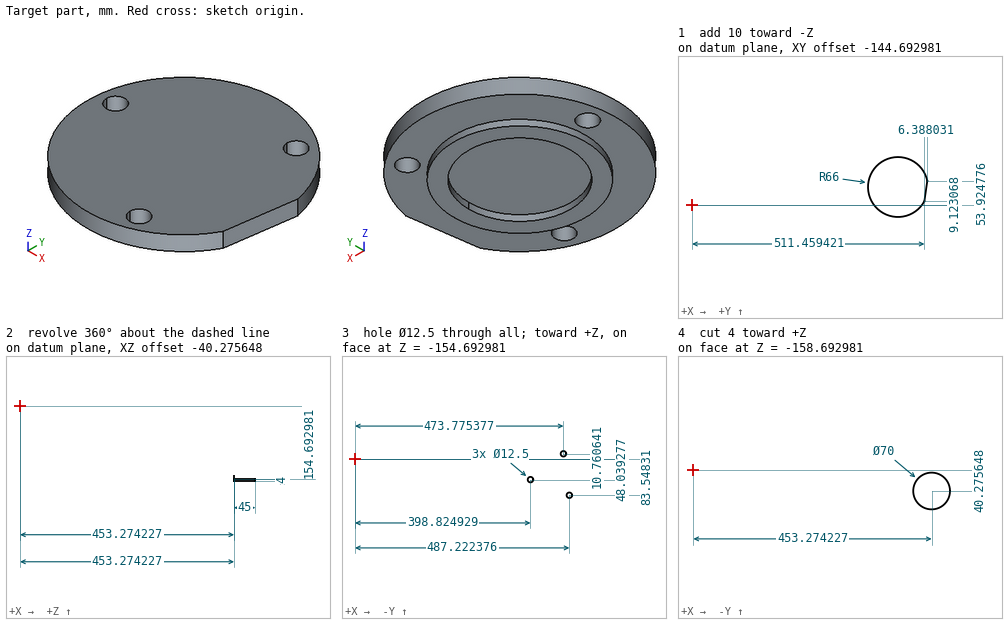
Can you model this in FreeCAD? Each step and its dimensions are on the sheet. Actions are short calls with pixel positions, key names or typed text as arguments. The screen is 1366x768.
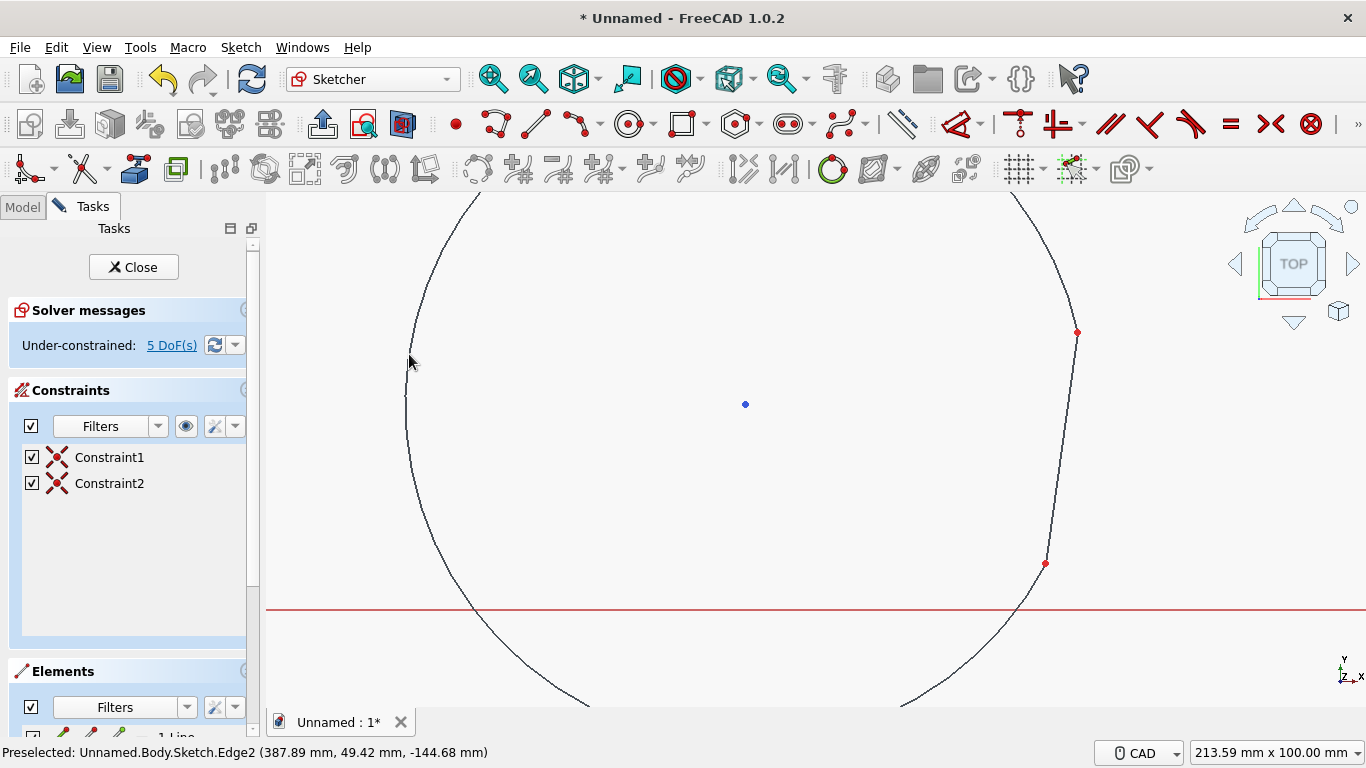
click(409, 358)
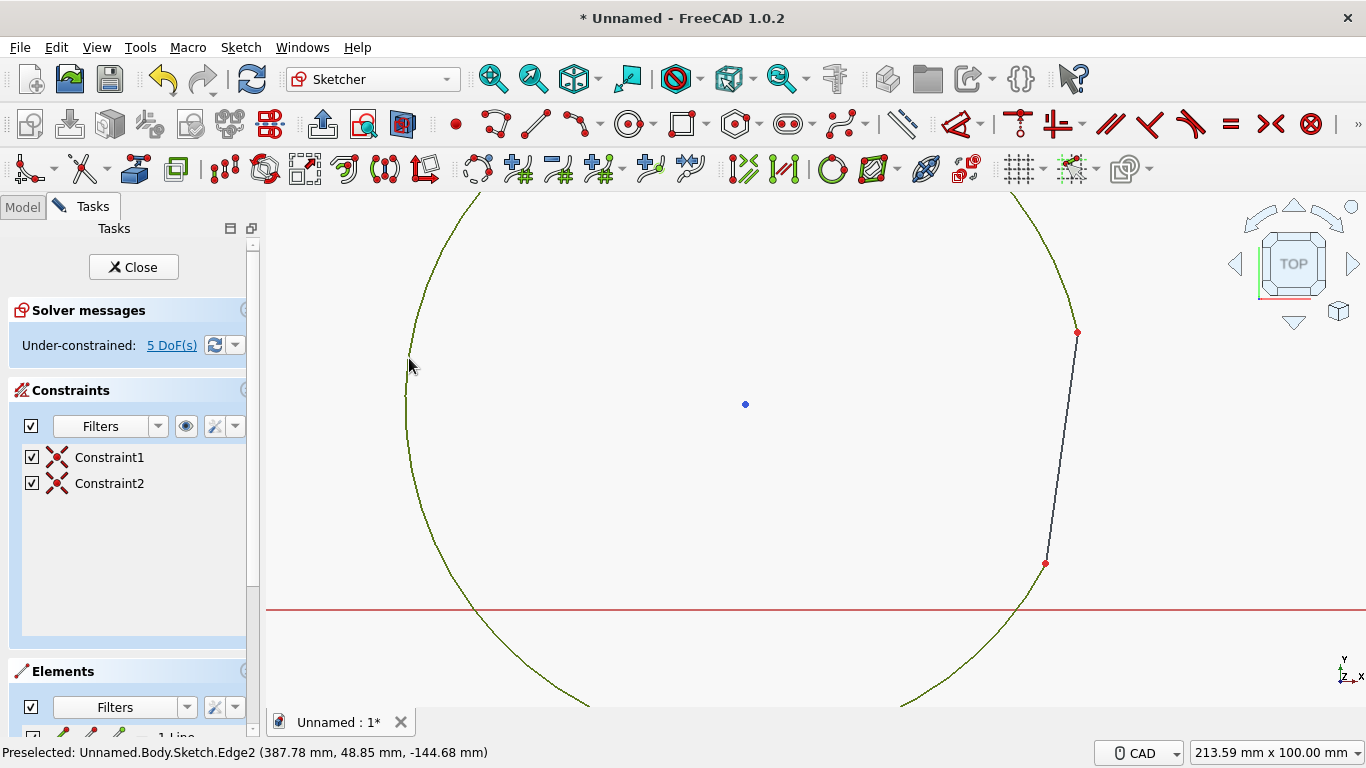
click(982, 124)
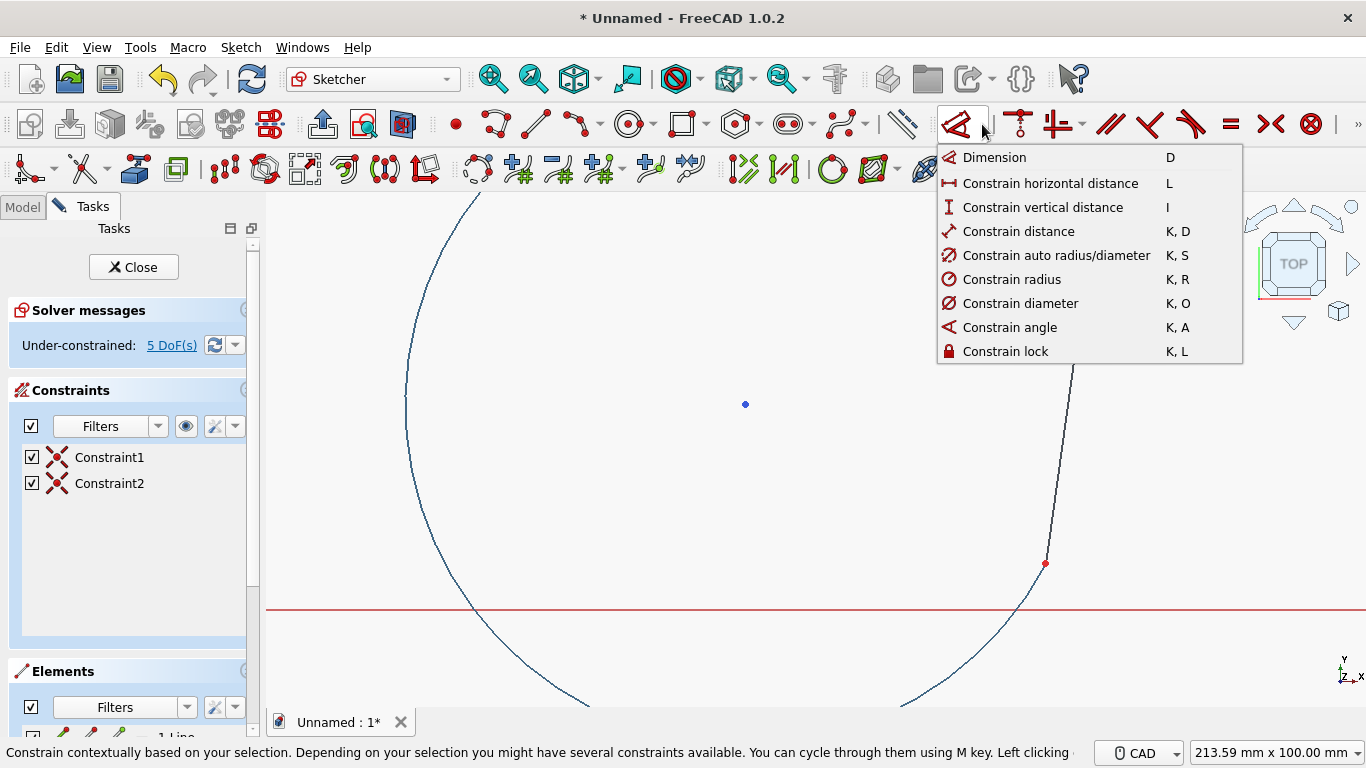
click(1090, 279)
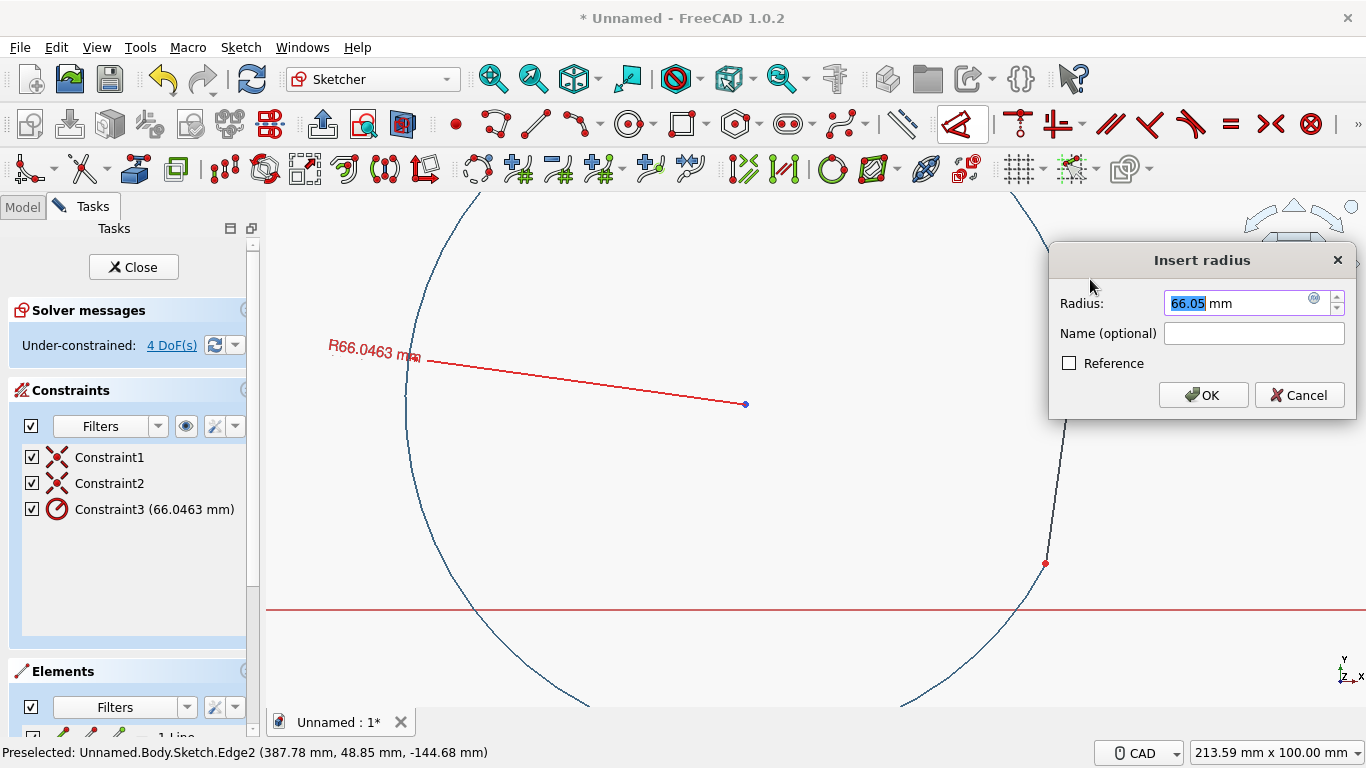
text(66)
key(Return)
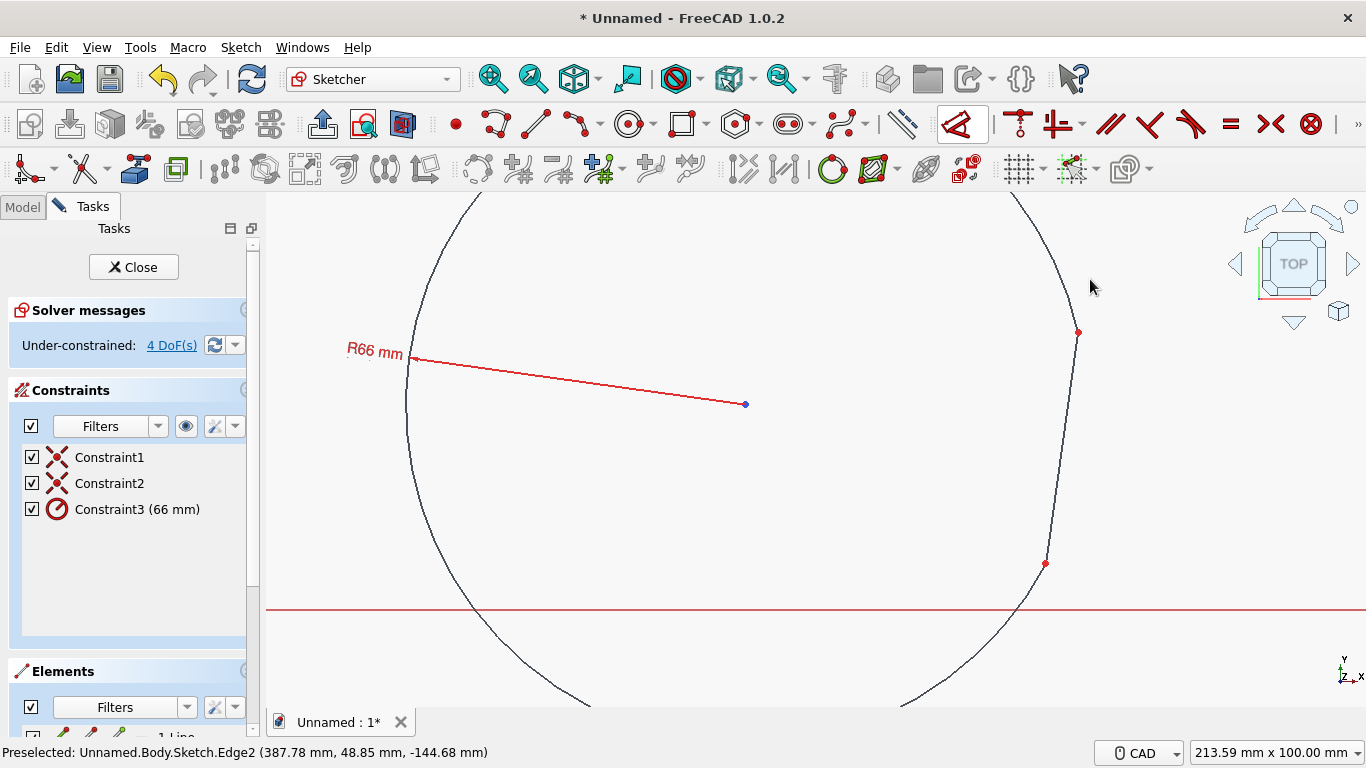
click(1046, 564)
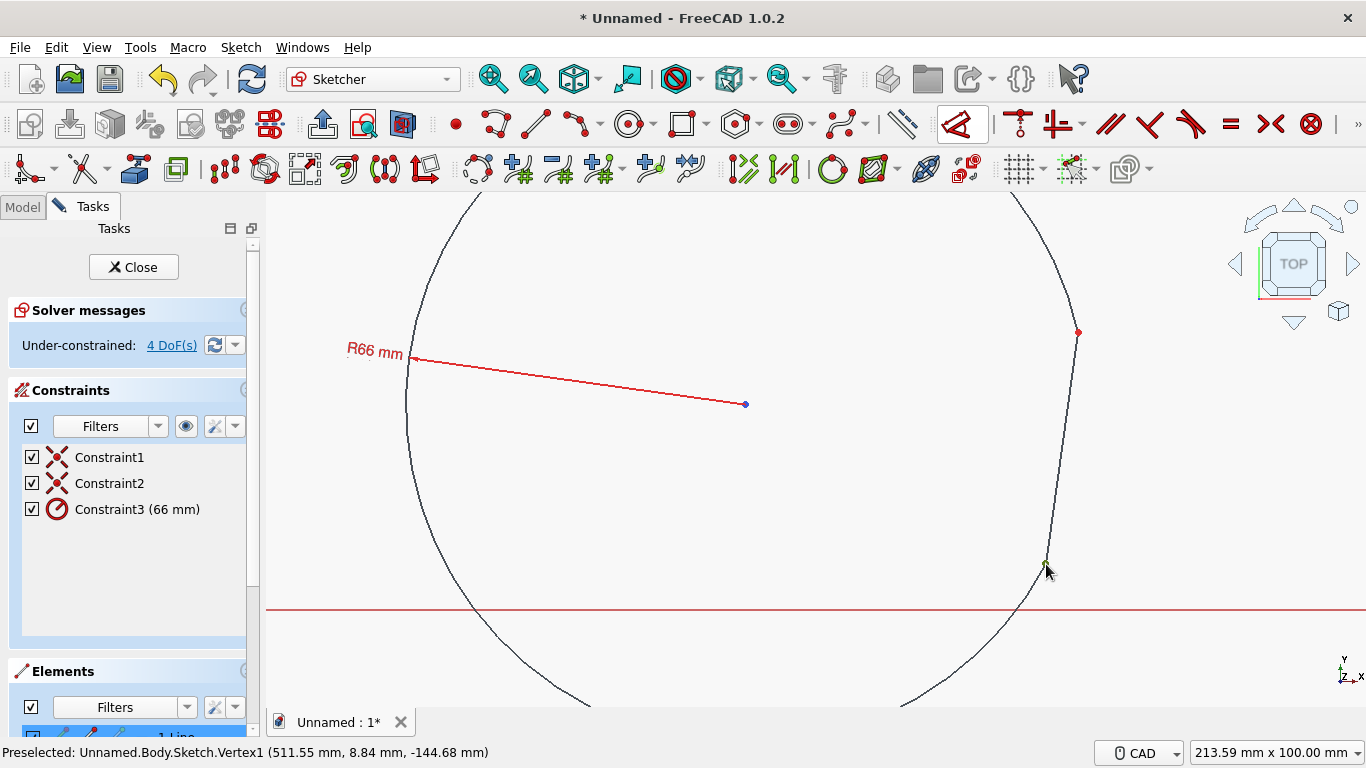
key(i)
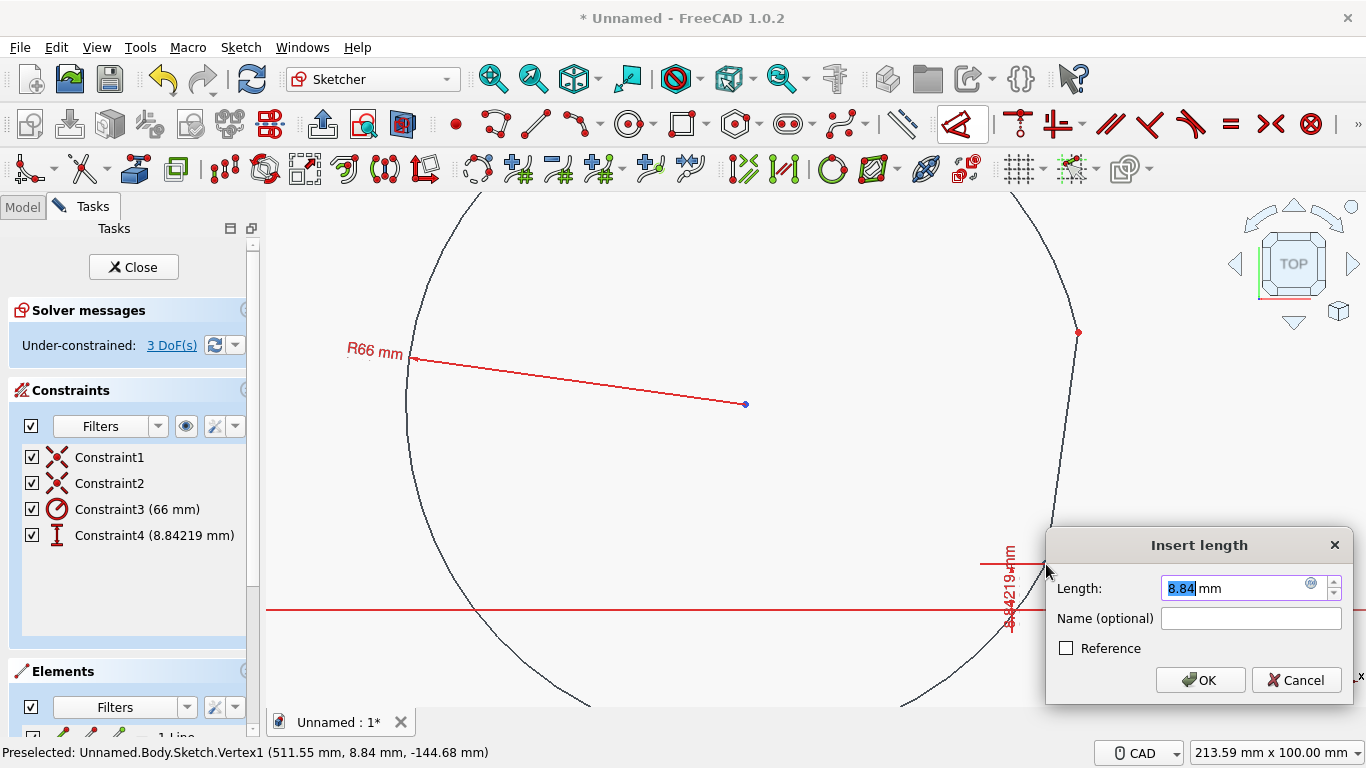
text(9.123068)
key(Return)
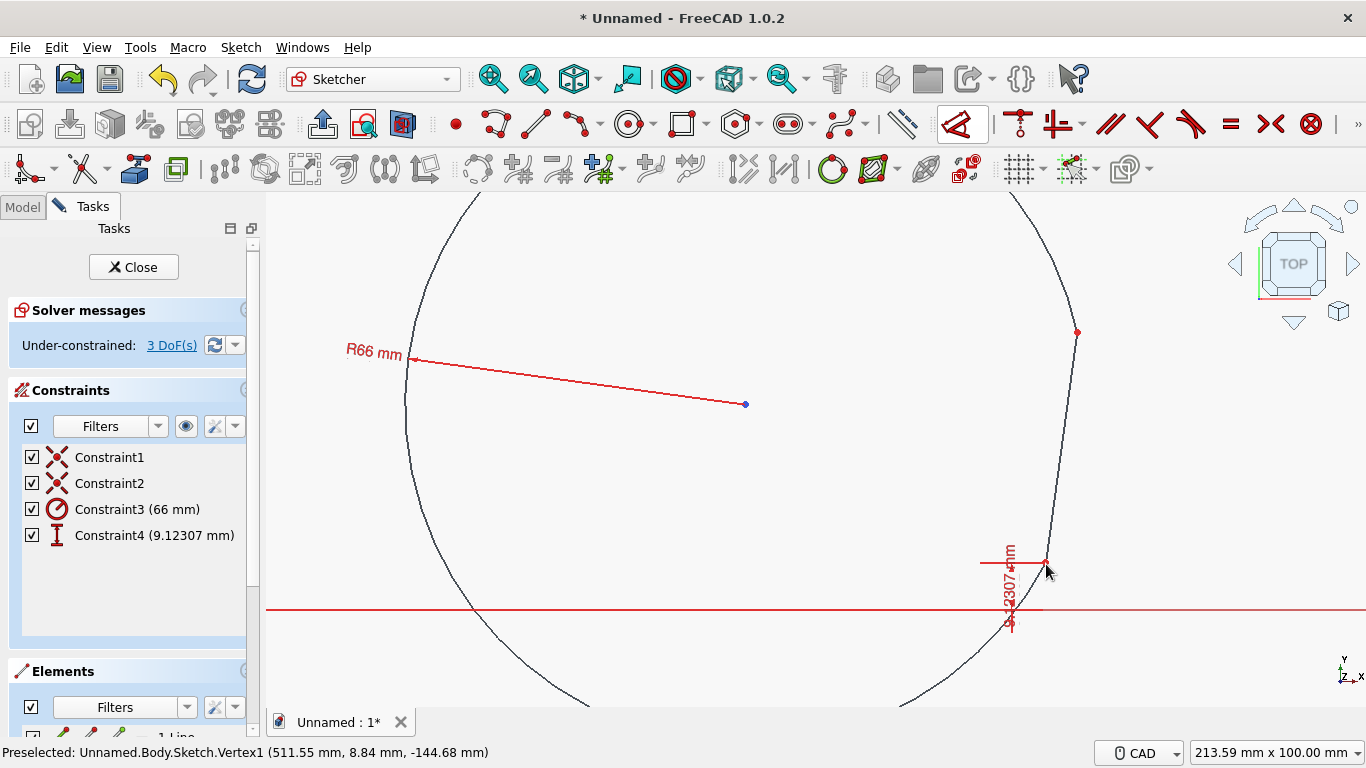
click(1055, 494)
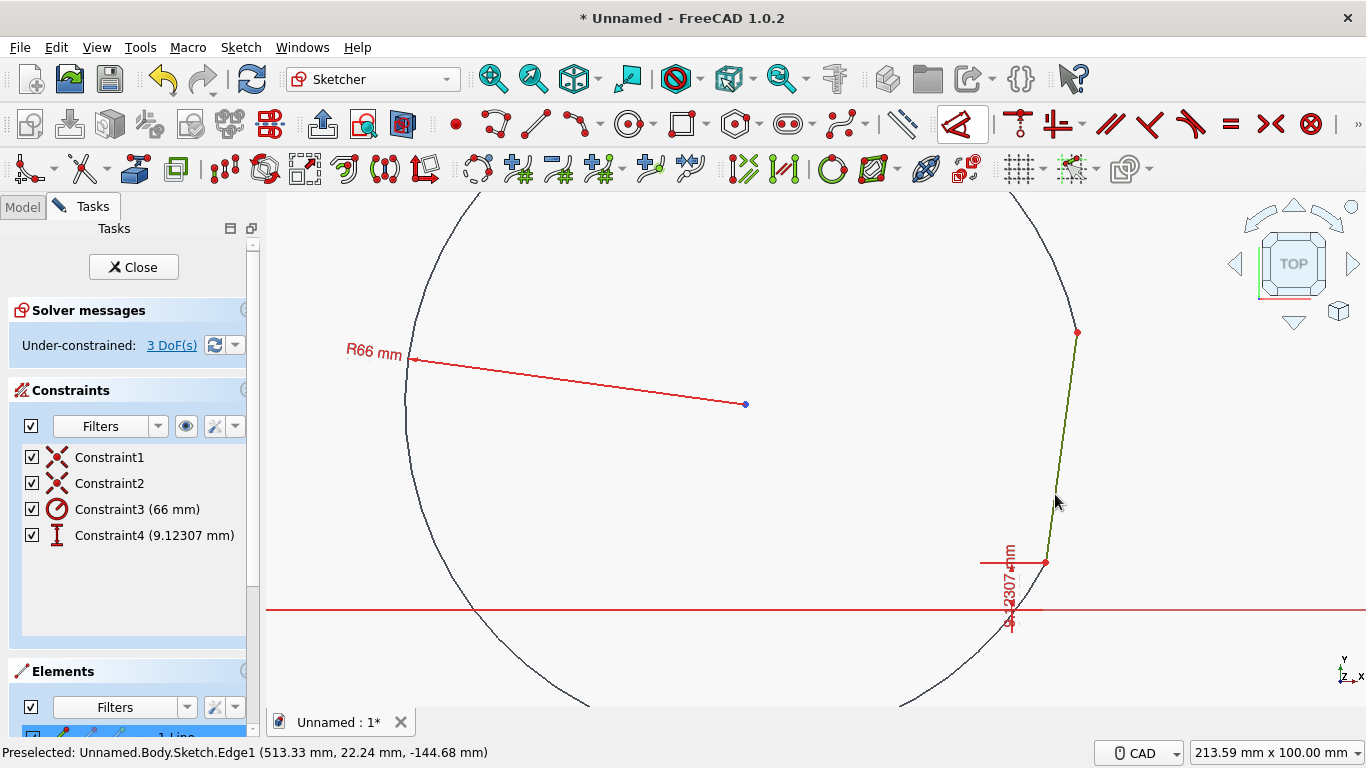
key(l)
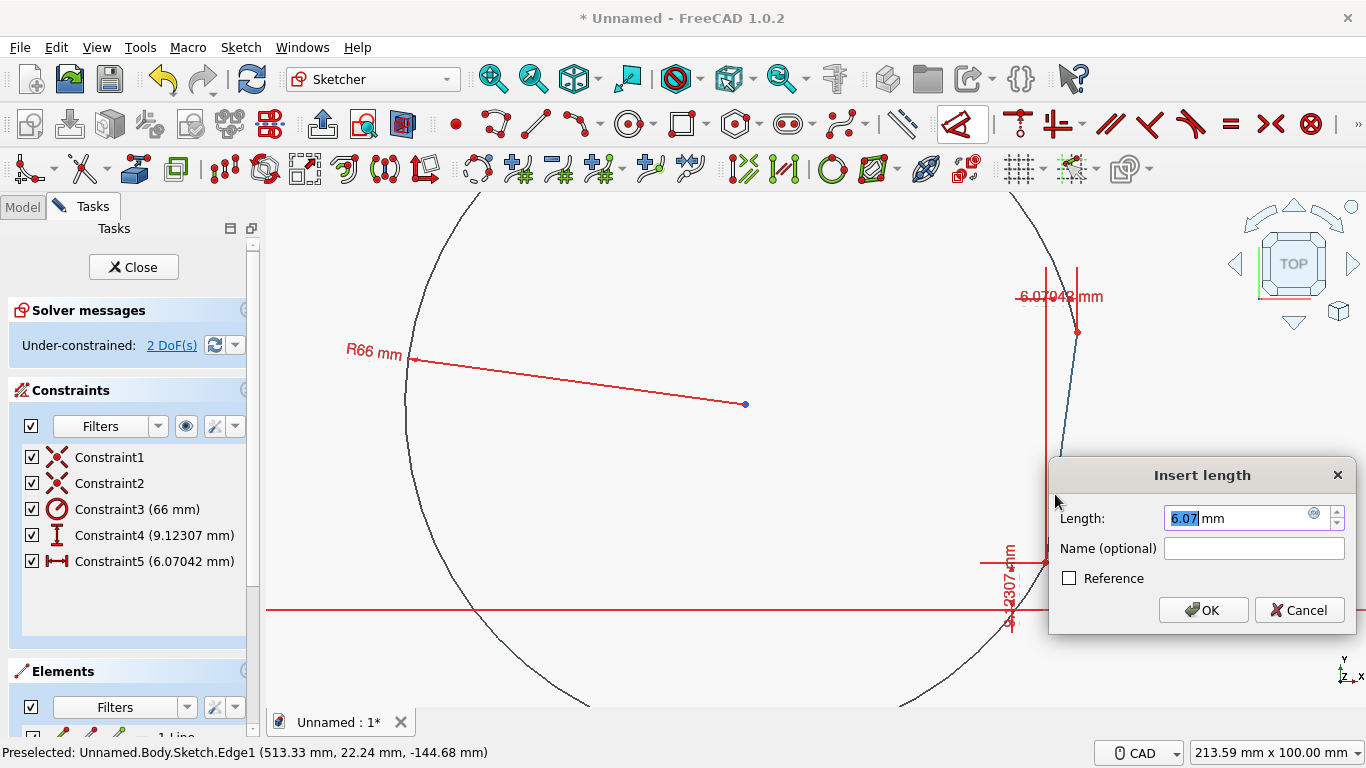
text(6.388031)
key(Return)